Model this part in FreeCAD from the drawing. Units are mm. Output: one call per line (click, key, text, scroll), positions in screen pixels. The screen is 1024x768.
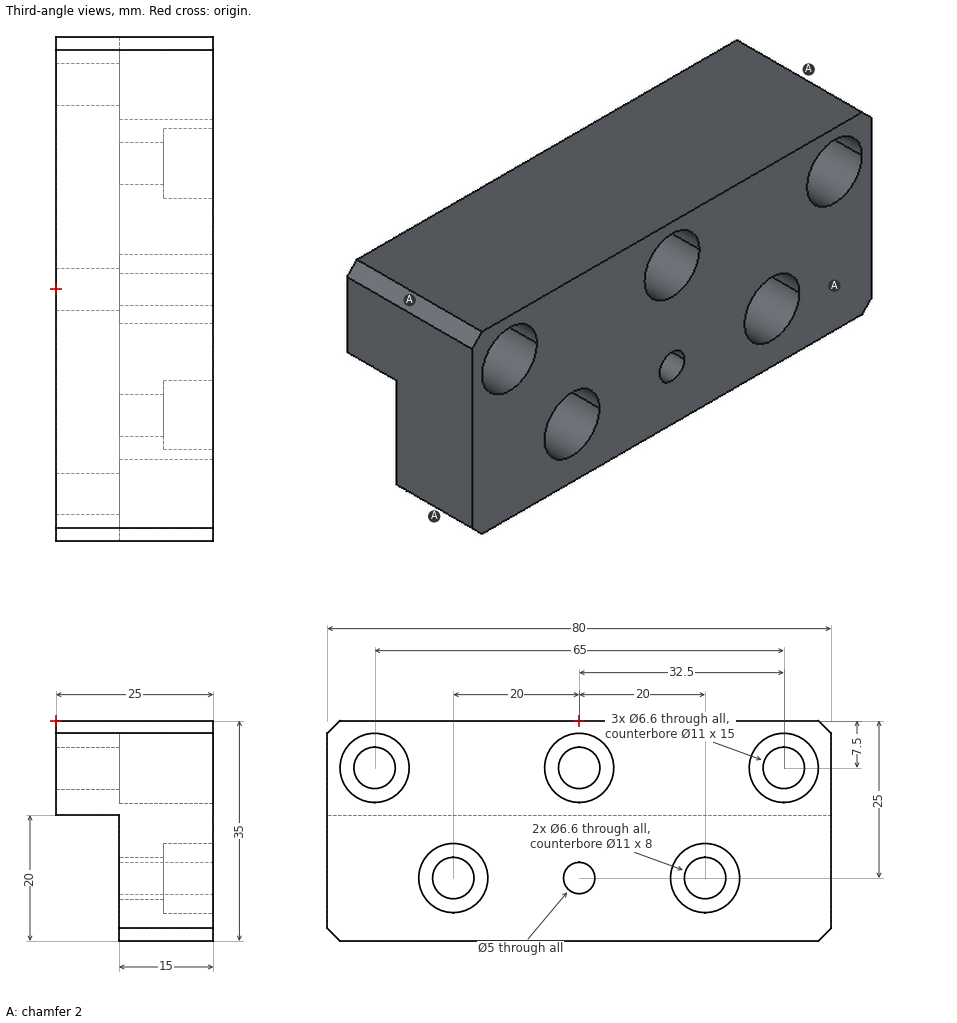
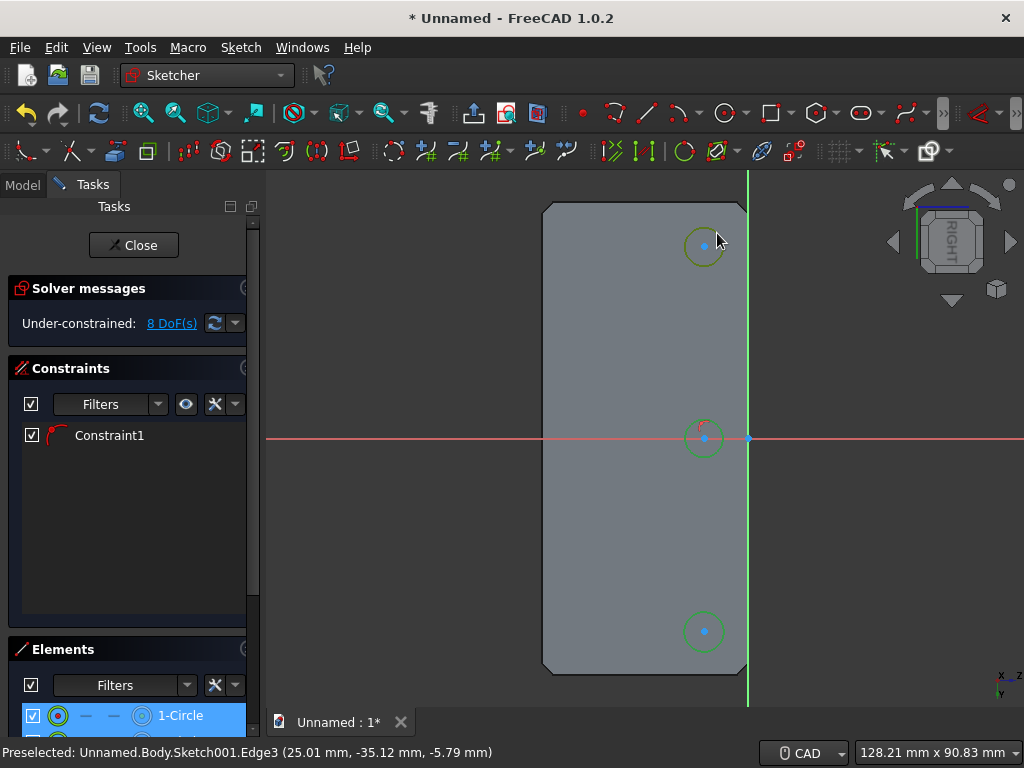
key(e)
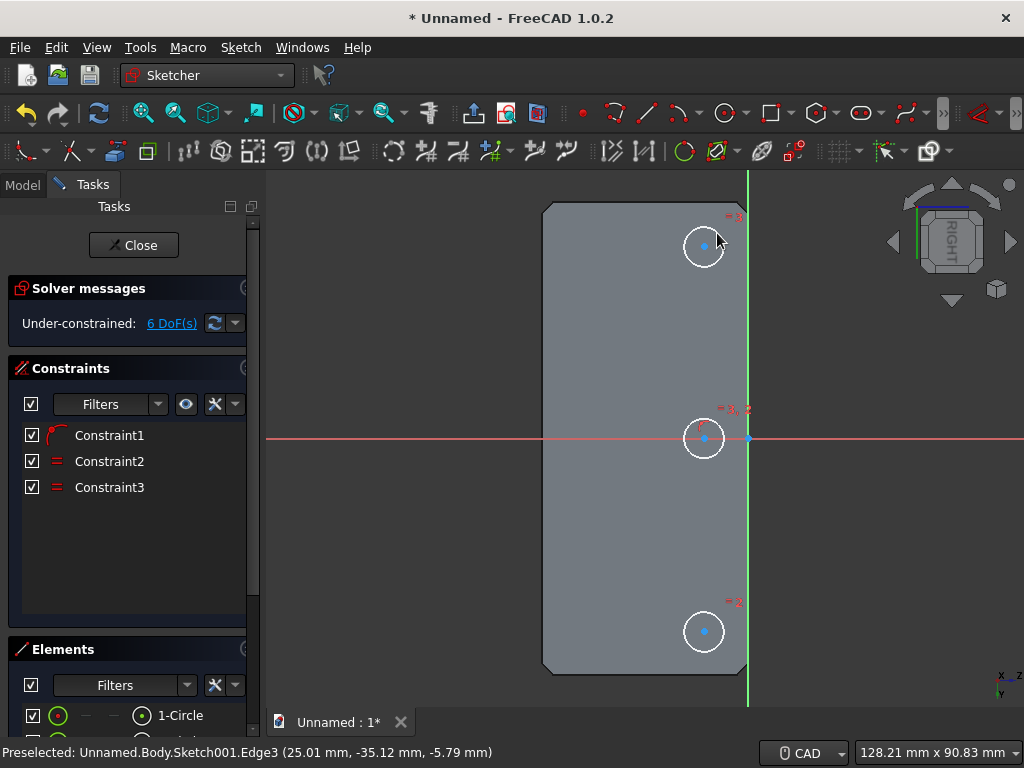
click(704, 632)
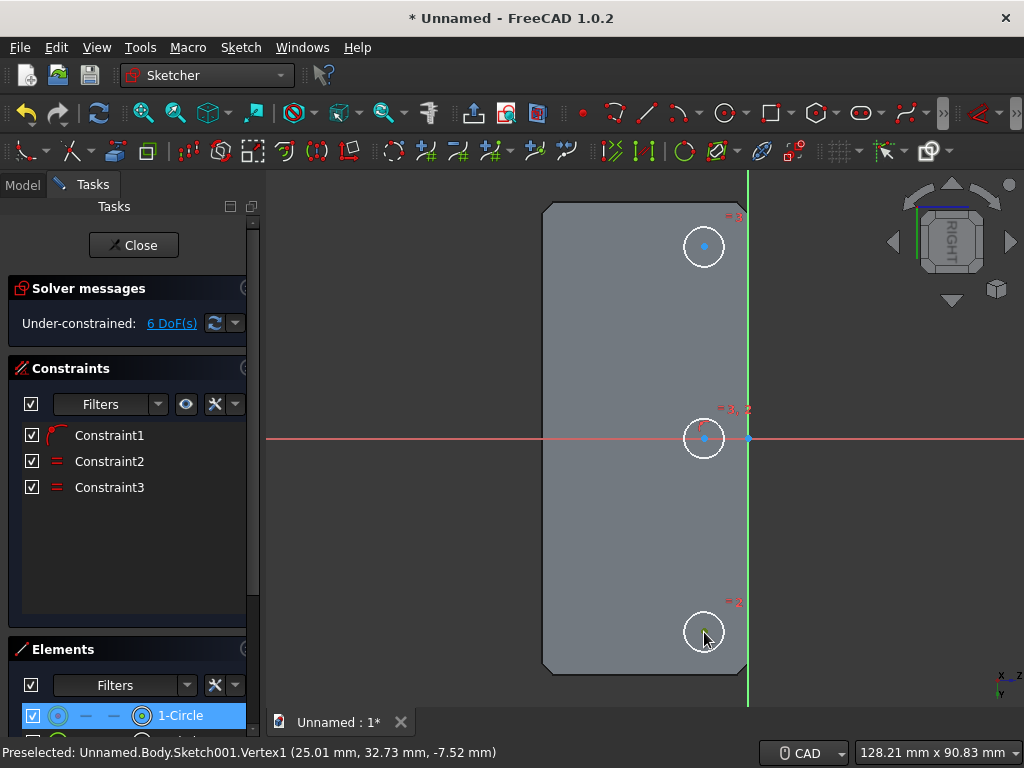
click(704, 438)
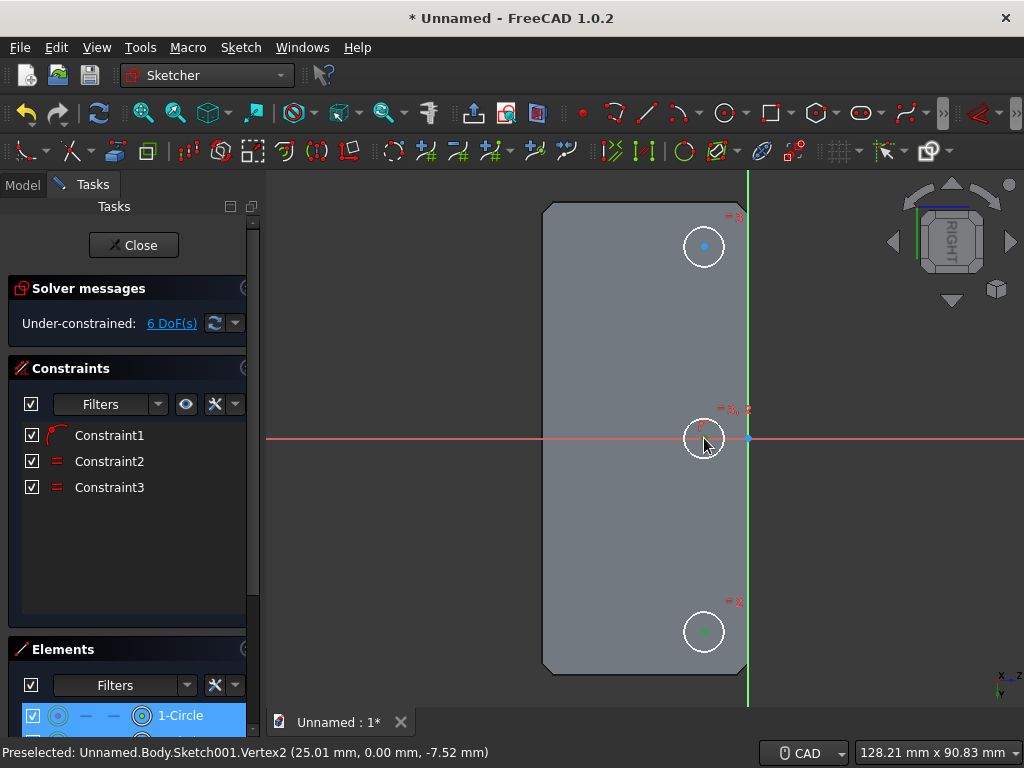
key(v)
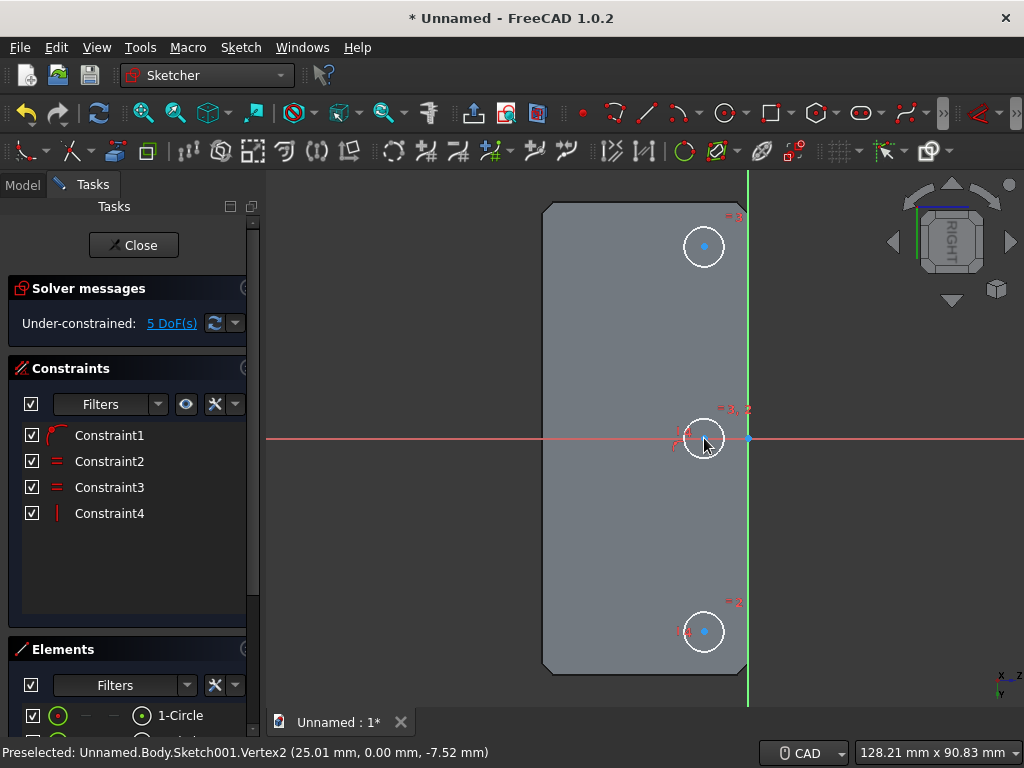
click(704, 438)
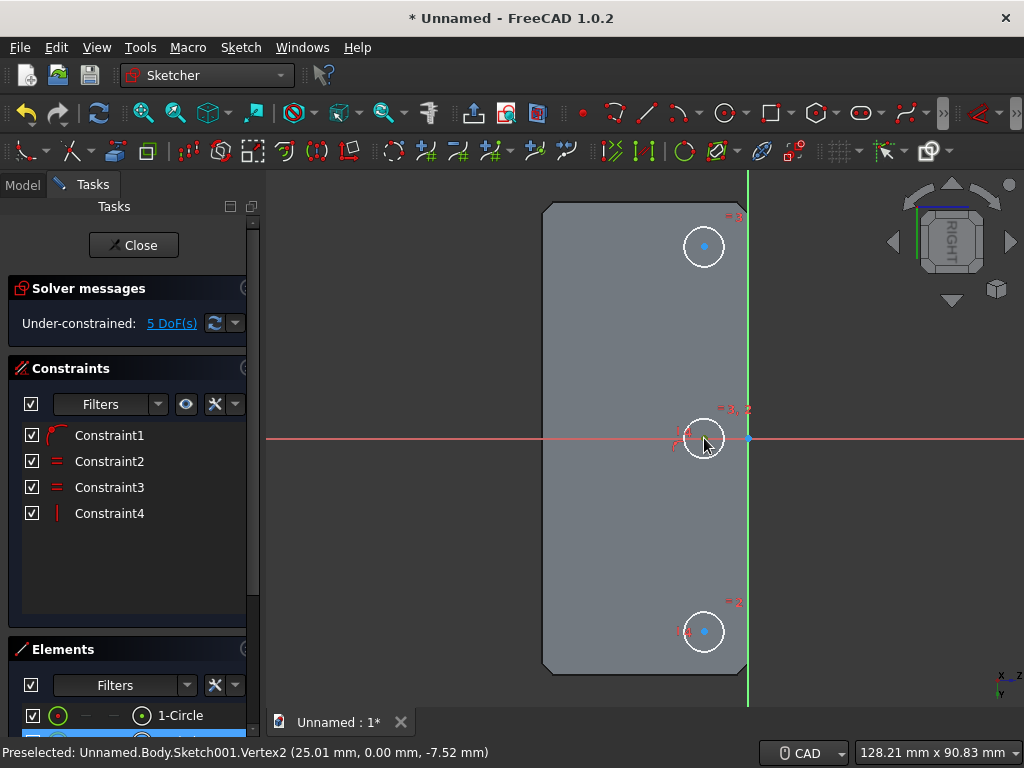
click(704, 247)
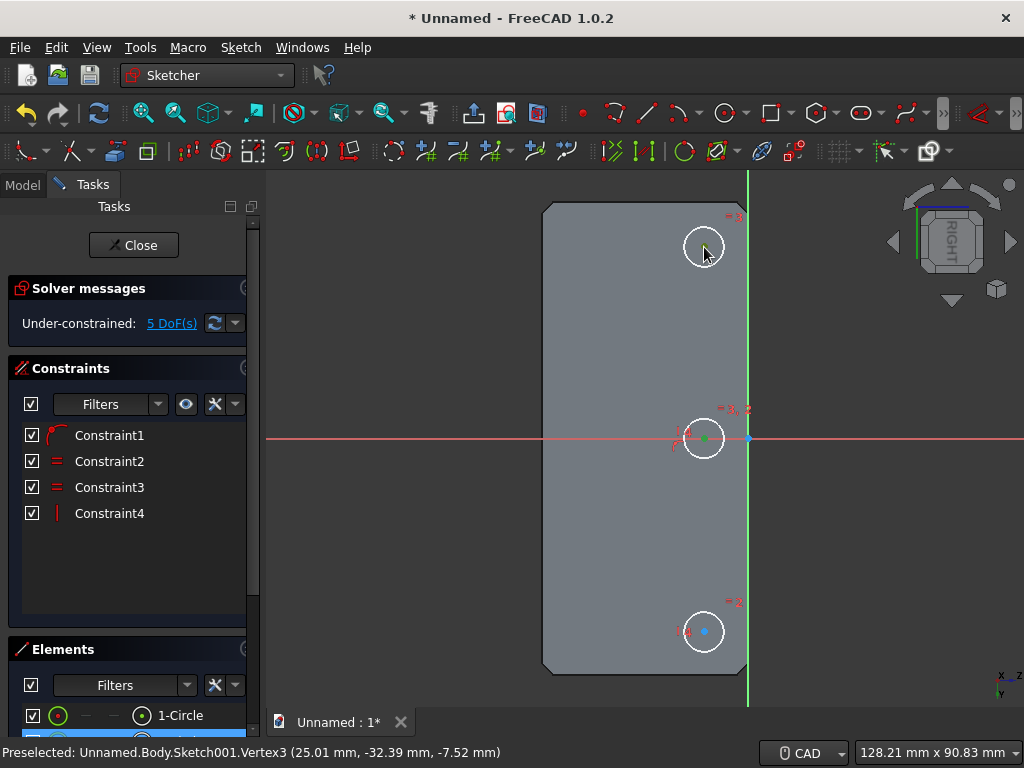
key(v)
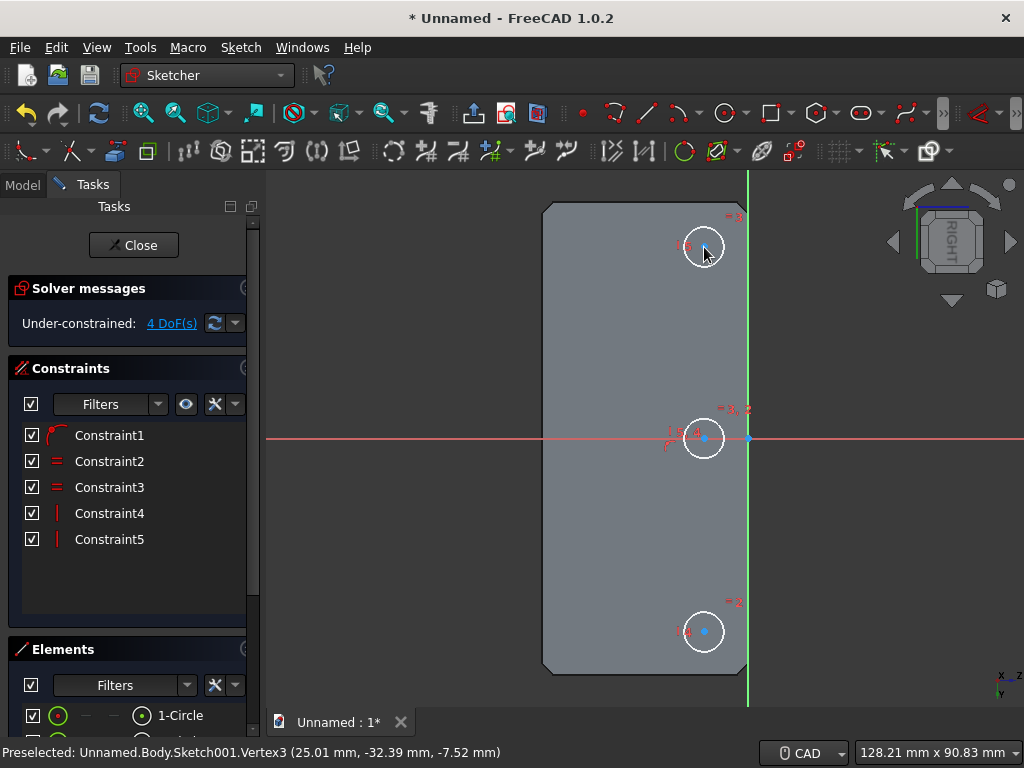
click(978, 114)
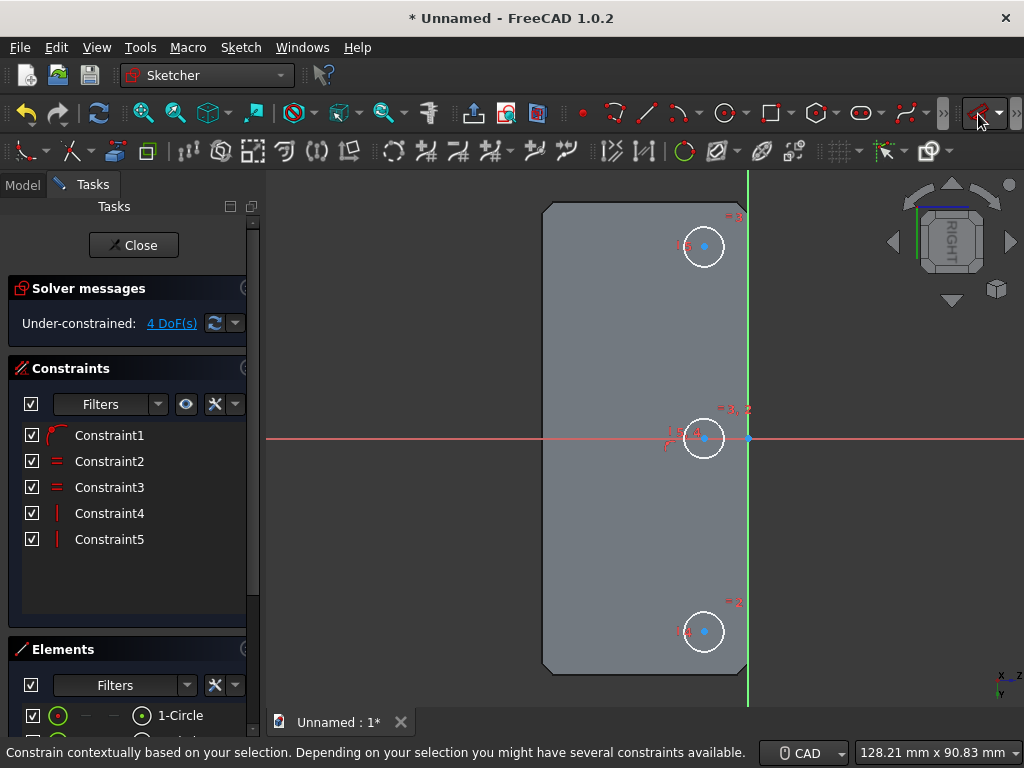
click(718, 618)
click(719, 582)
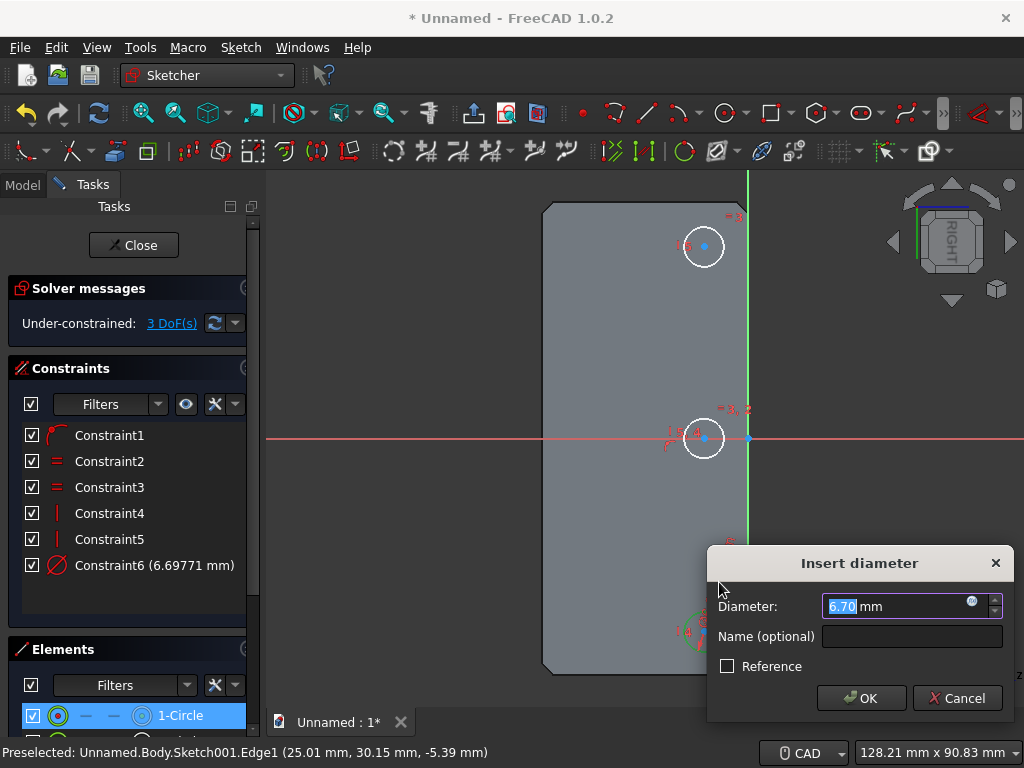
text(6.6)
key(Return)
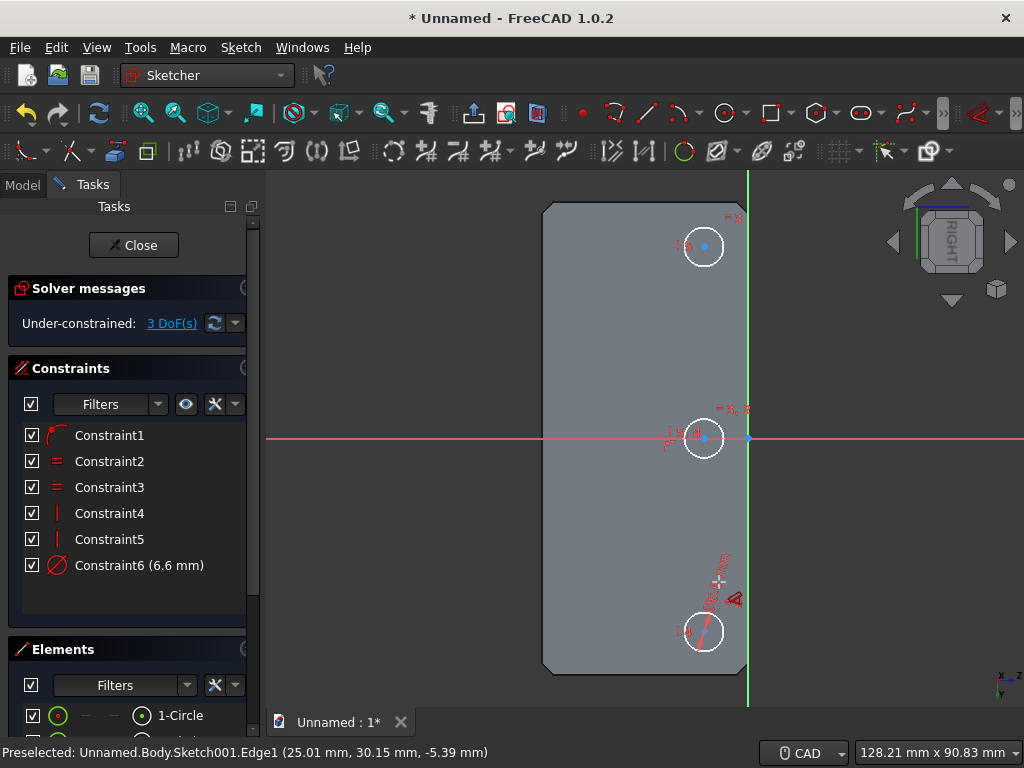
click(704, 632)
click(726, 666)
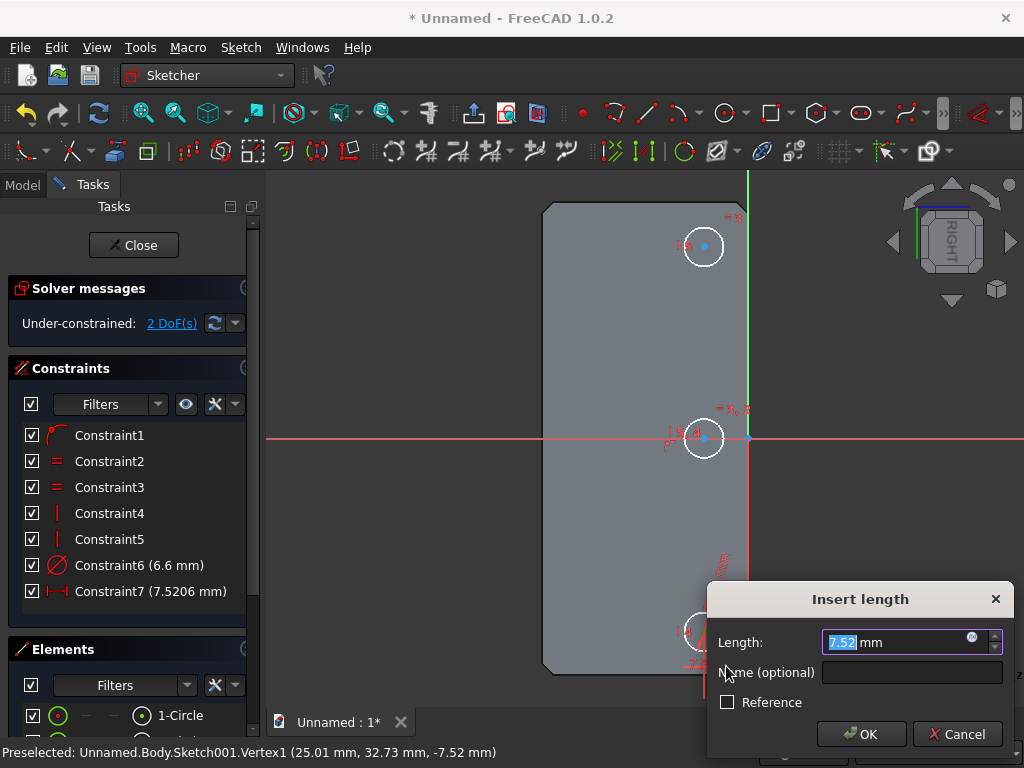
text(7.5)
key(Return)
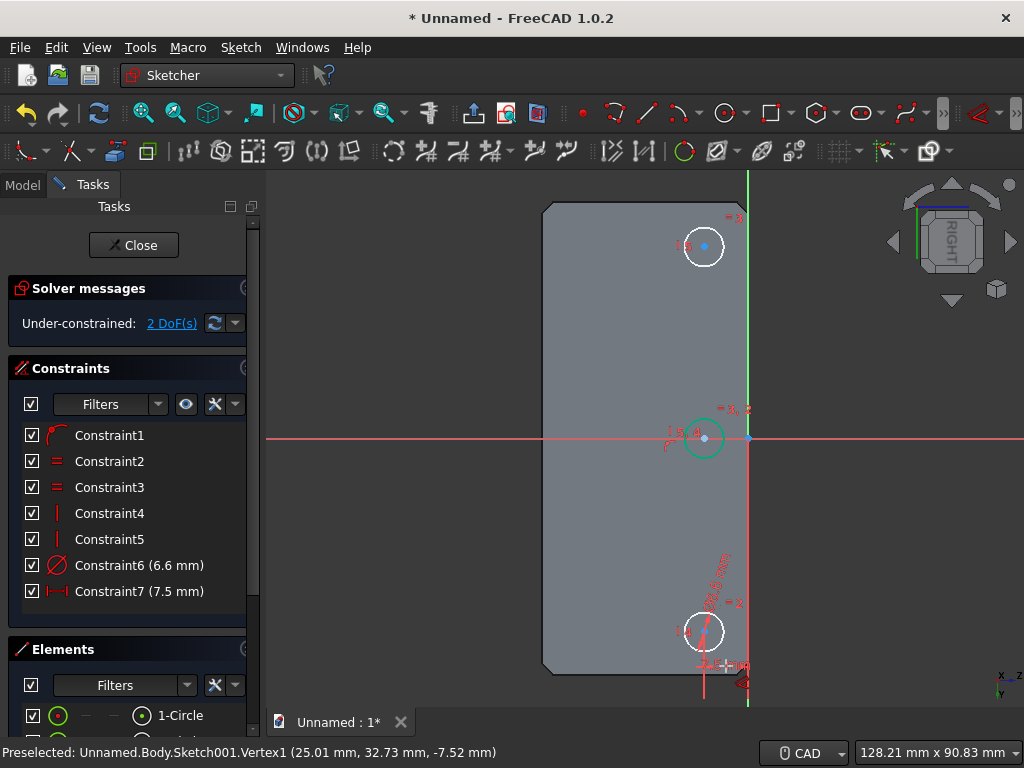
click(704, 632)